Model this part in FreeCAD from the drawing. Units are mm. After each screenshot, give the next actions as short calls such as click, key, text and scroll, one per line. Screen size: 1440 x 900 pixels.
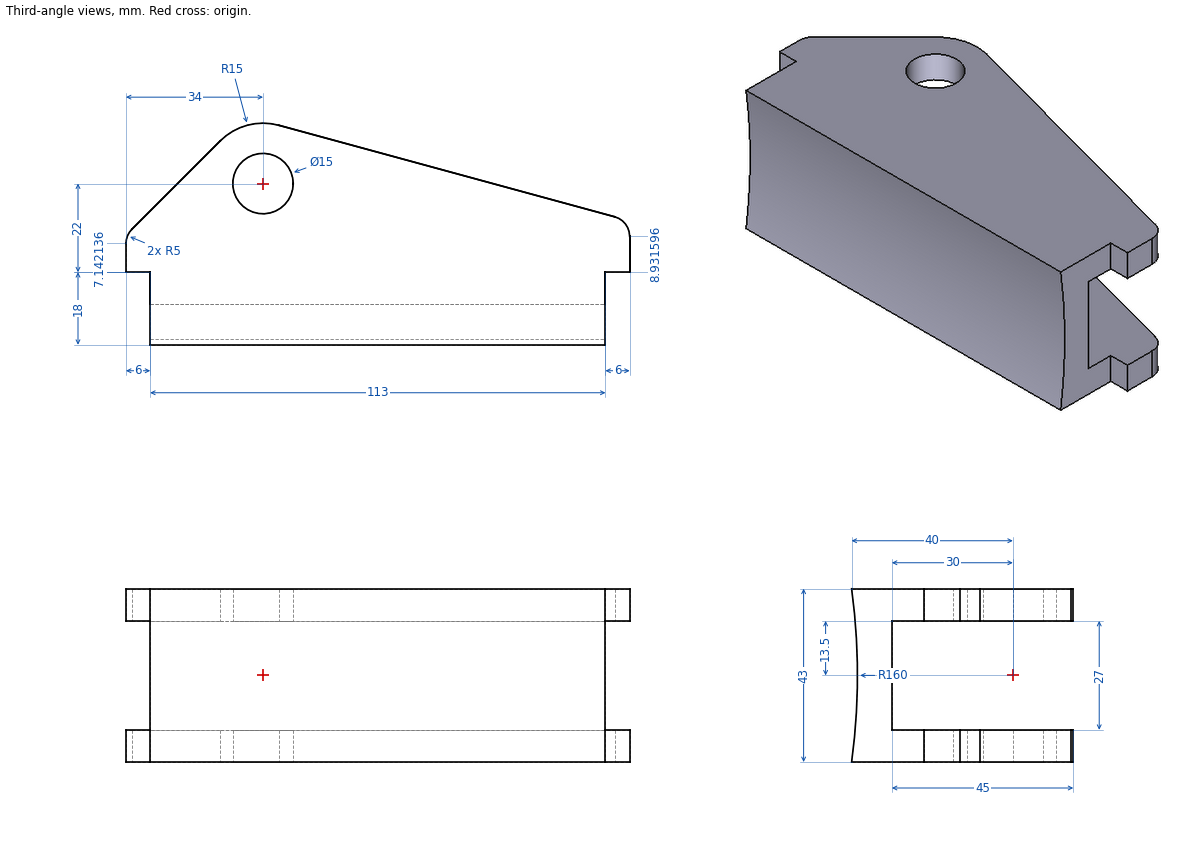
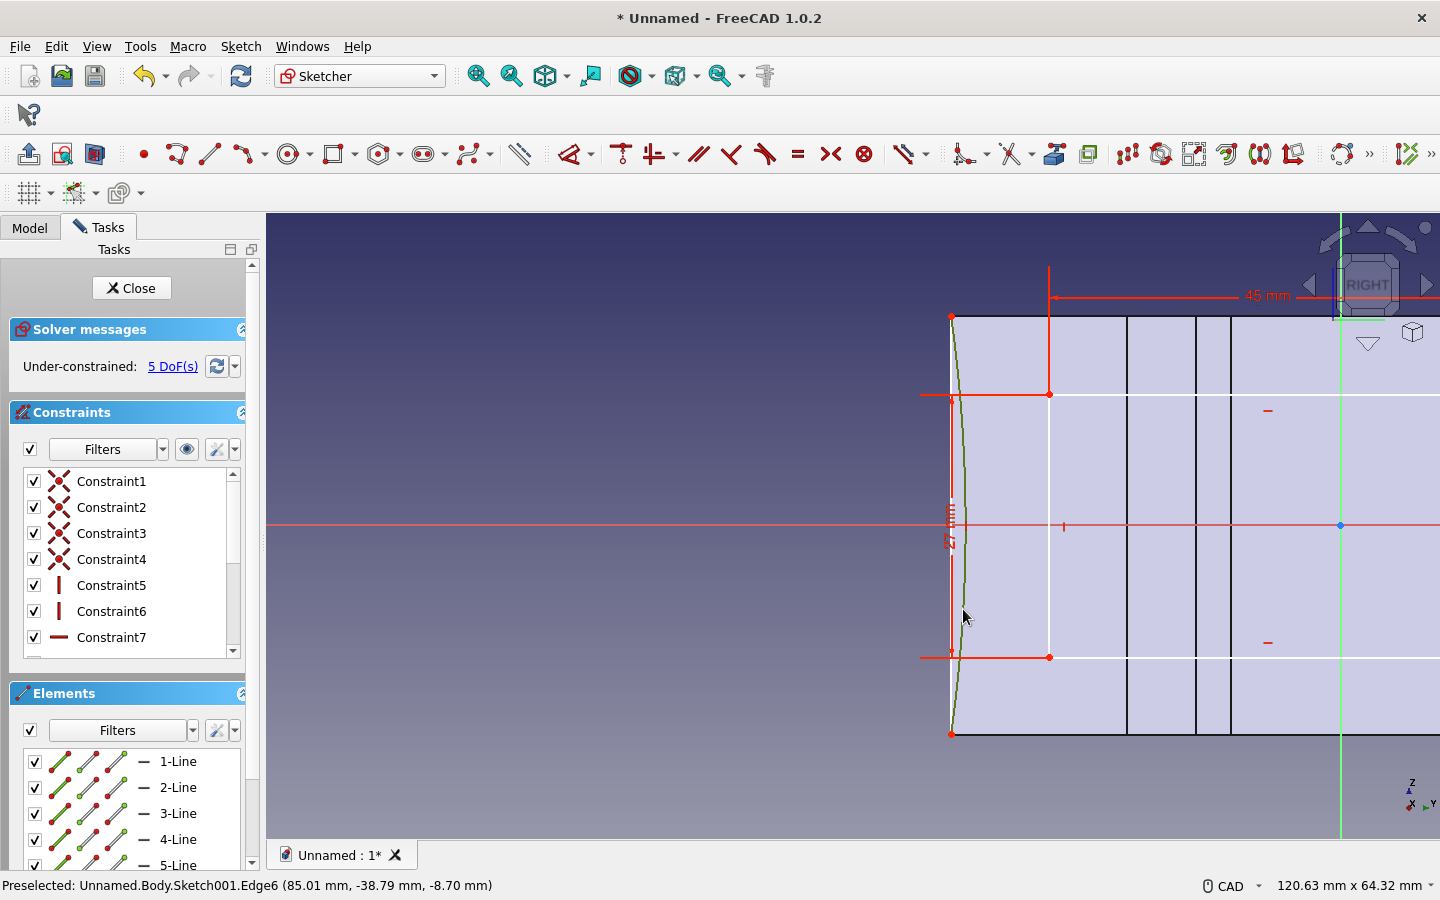
key(k)
key(r)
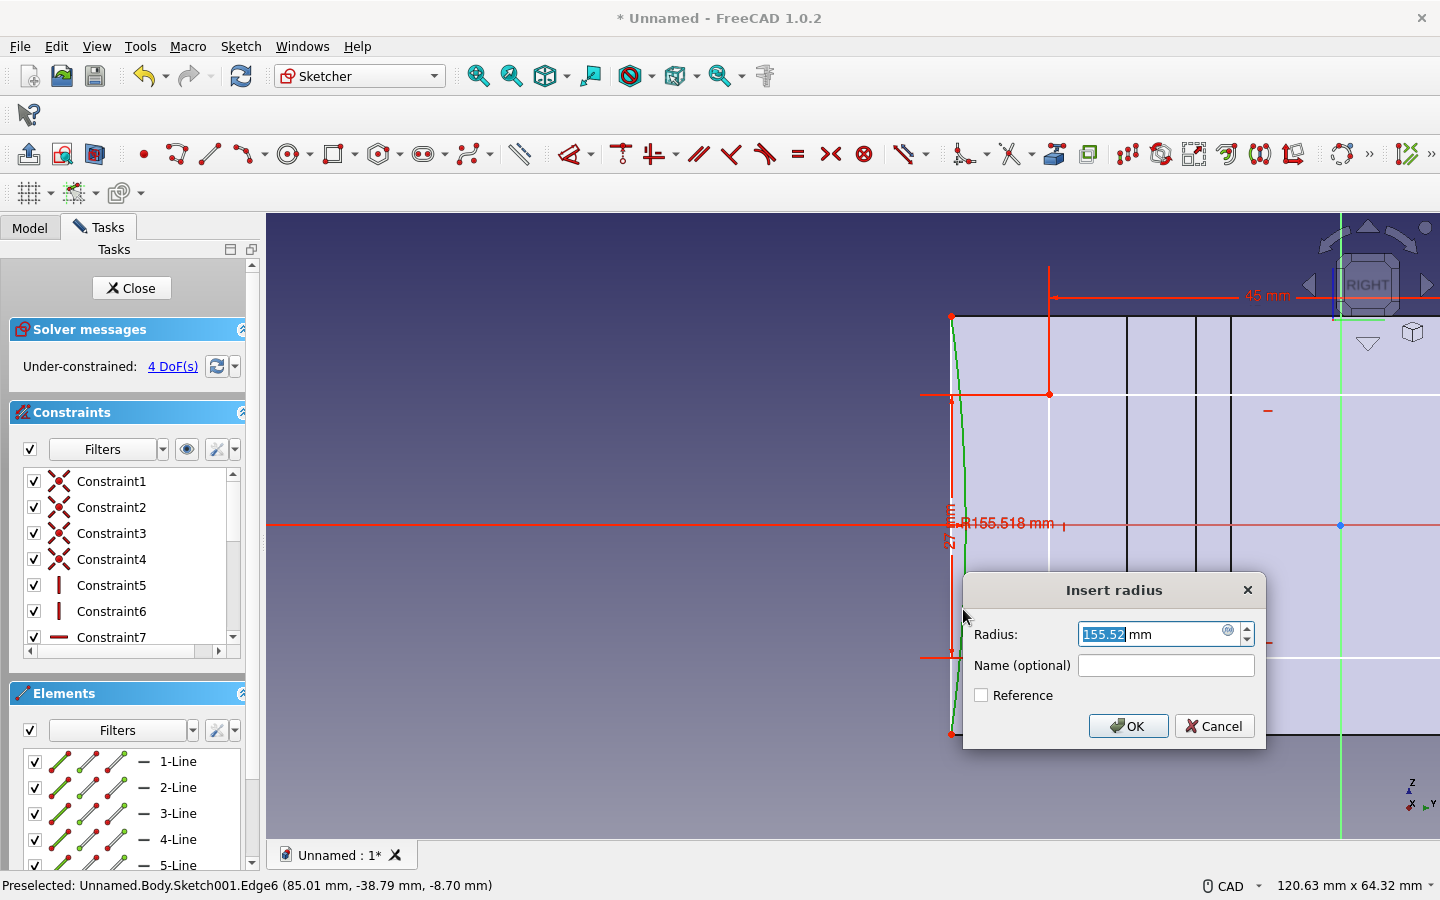
text(160)
key(Return)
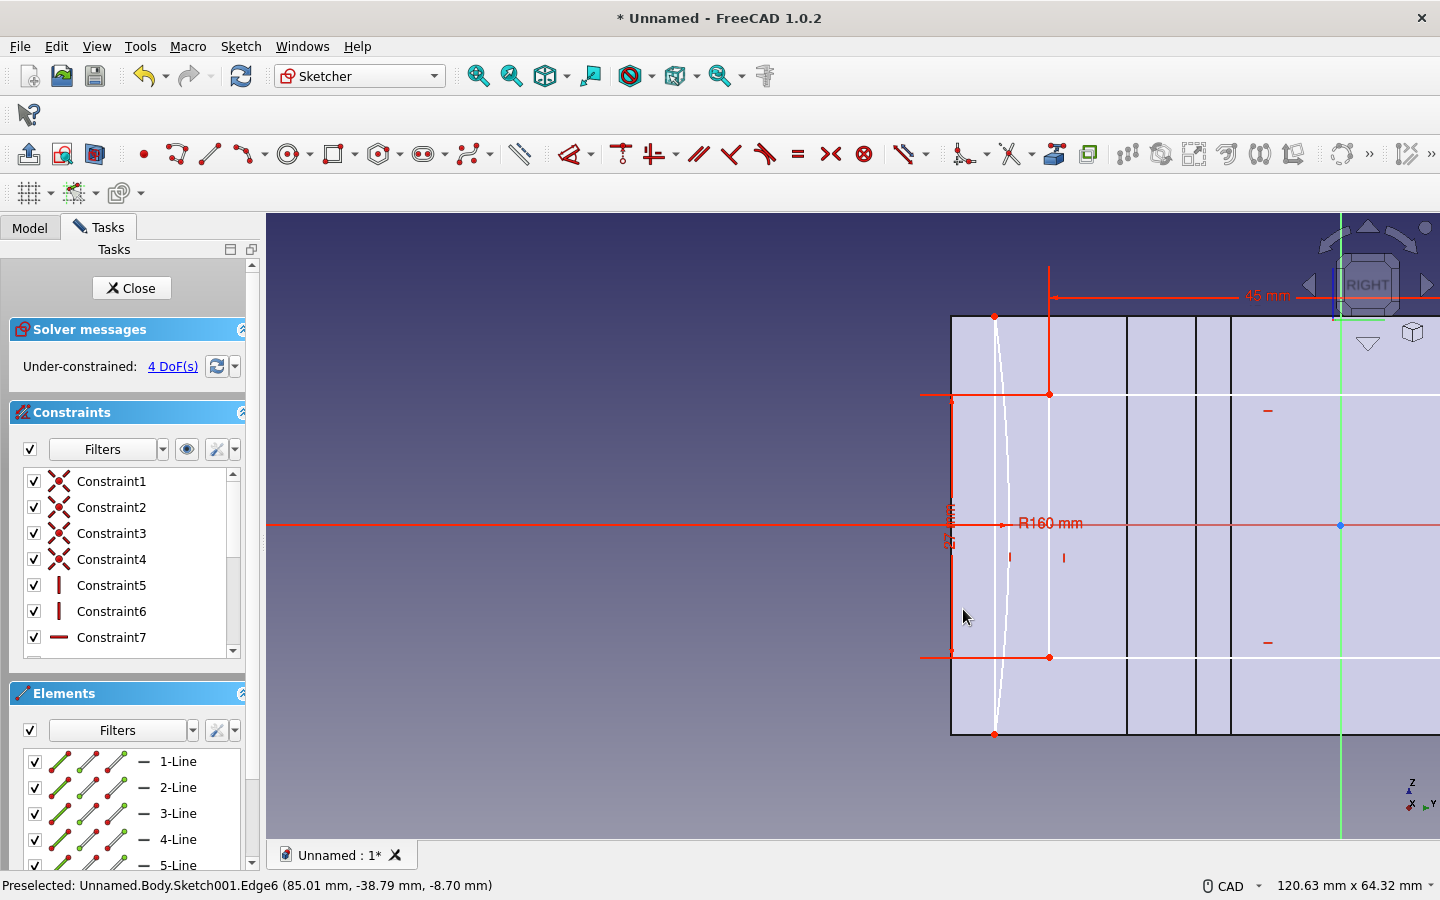
click(995, 442)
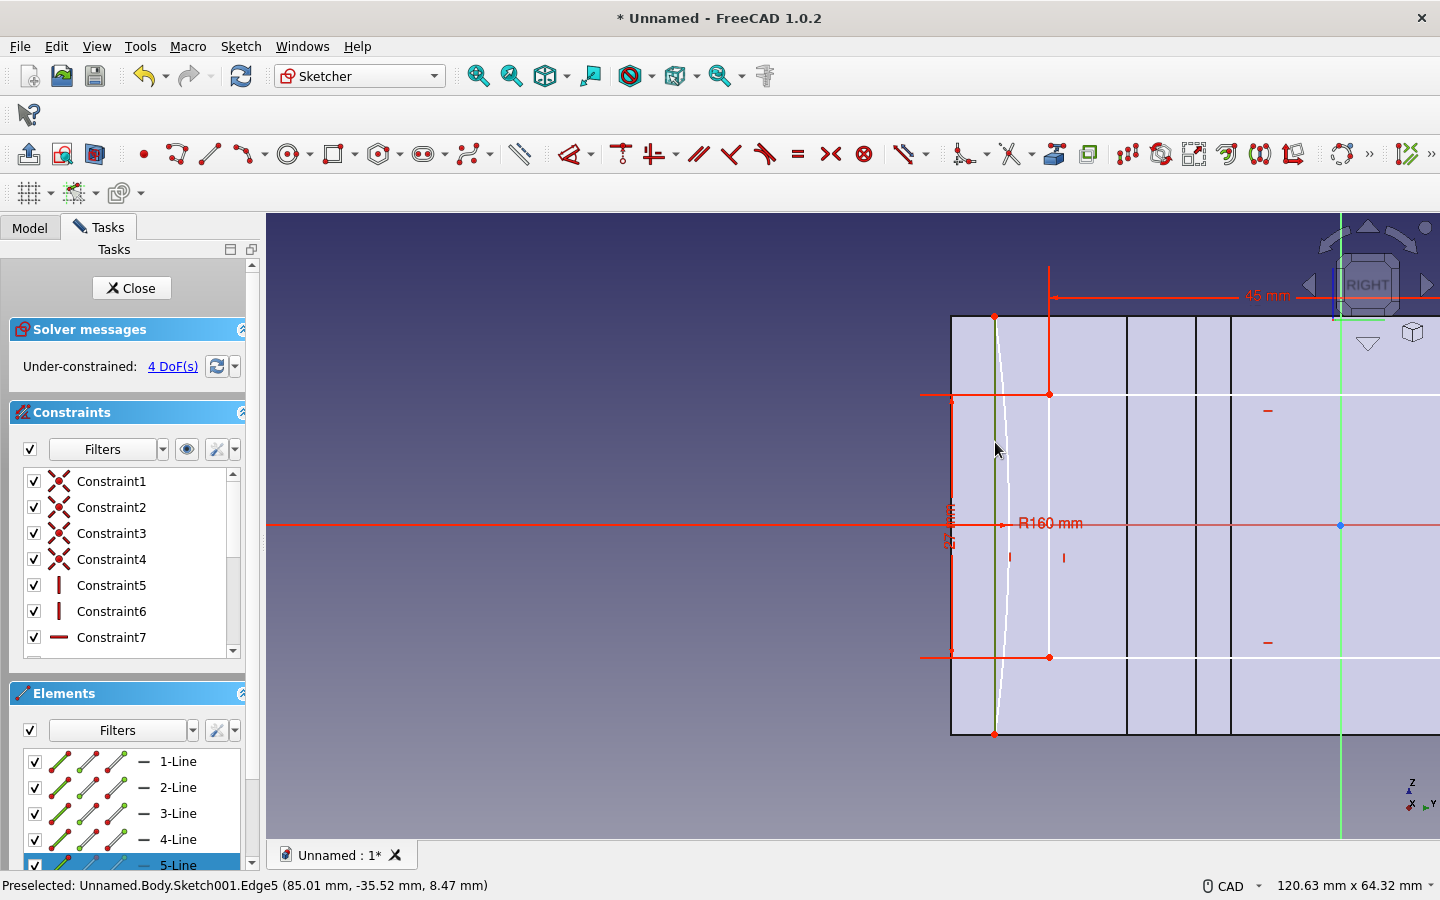
key(i)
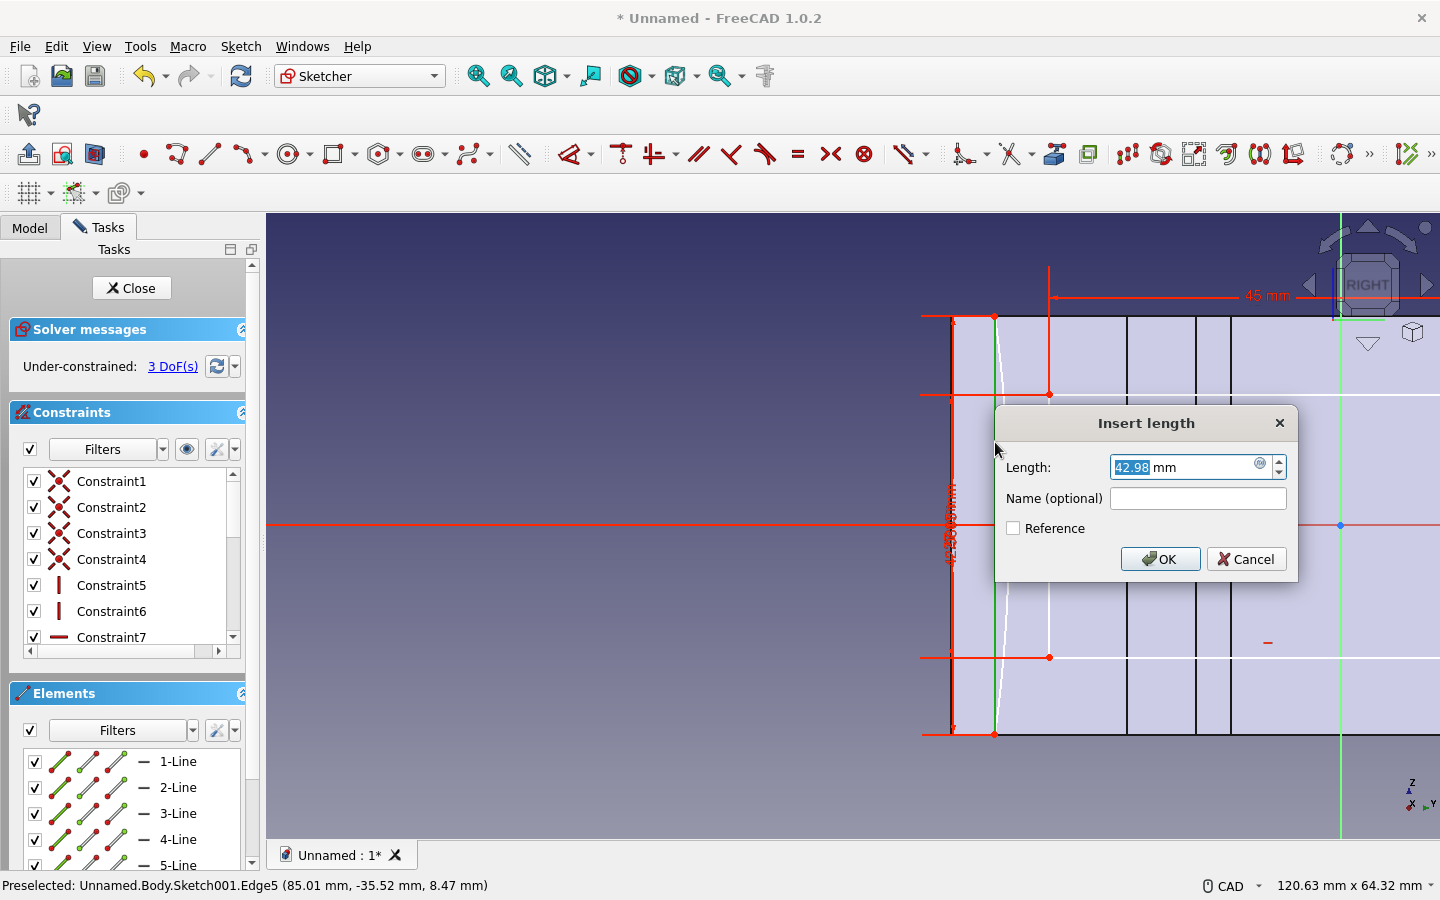
text(43)
key(Return)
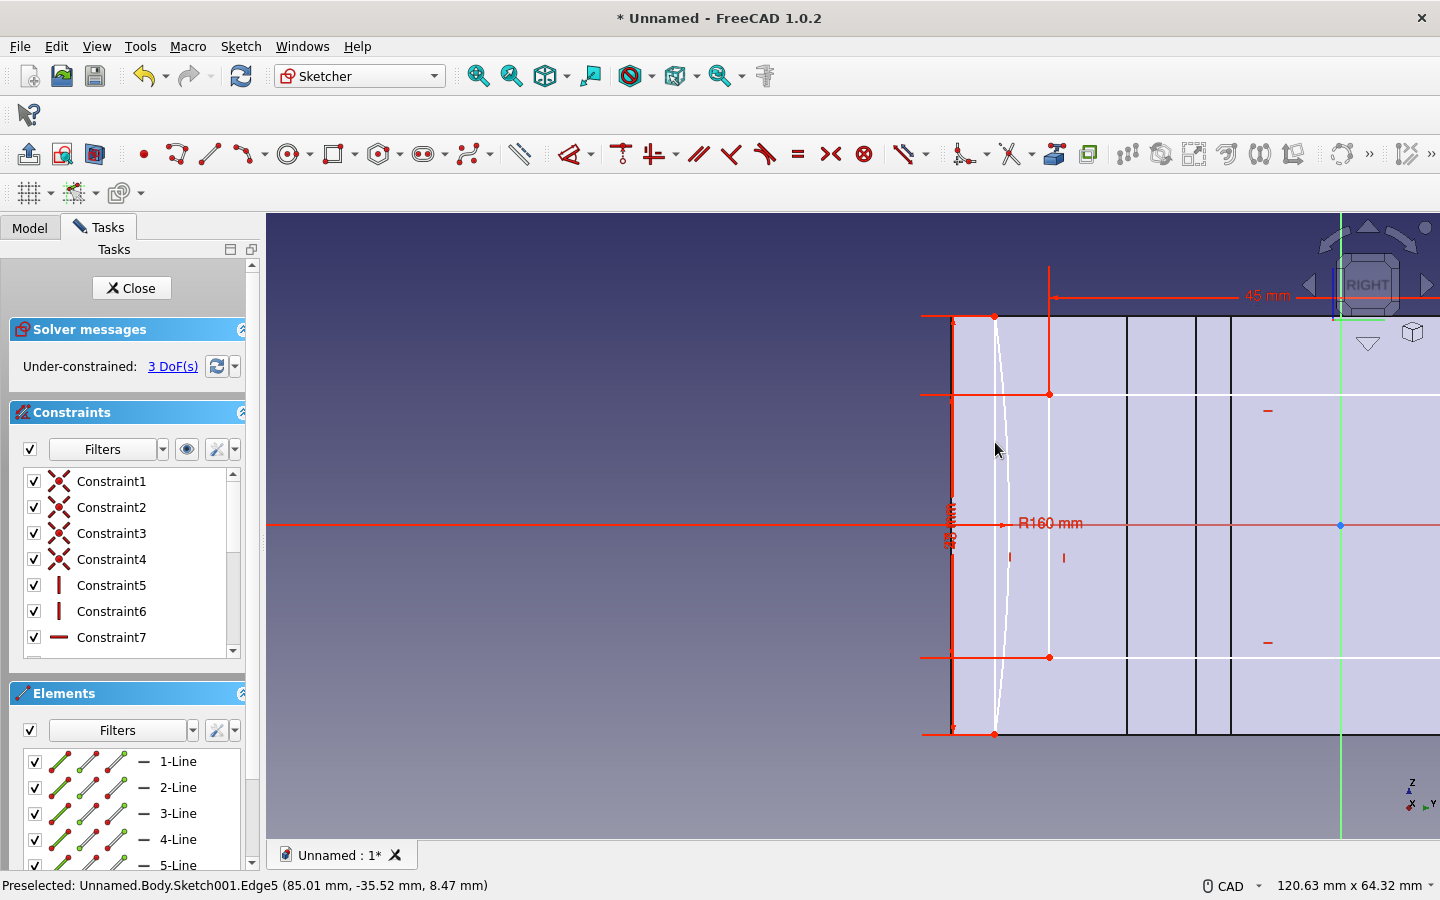
click(1049, 395)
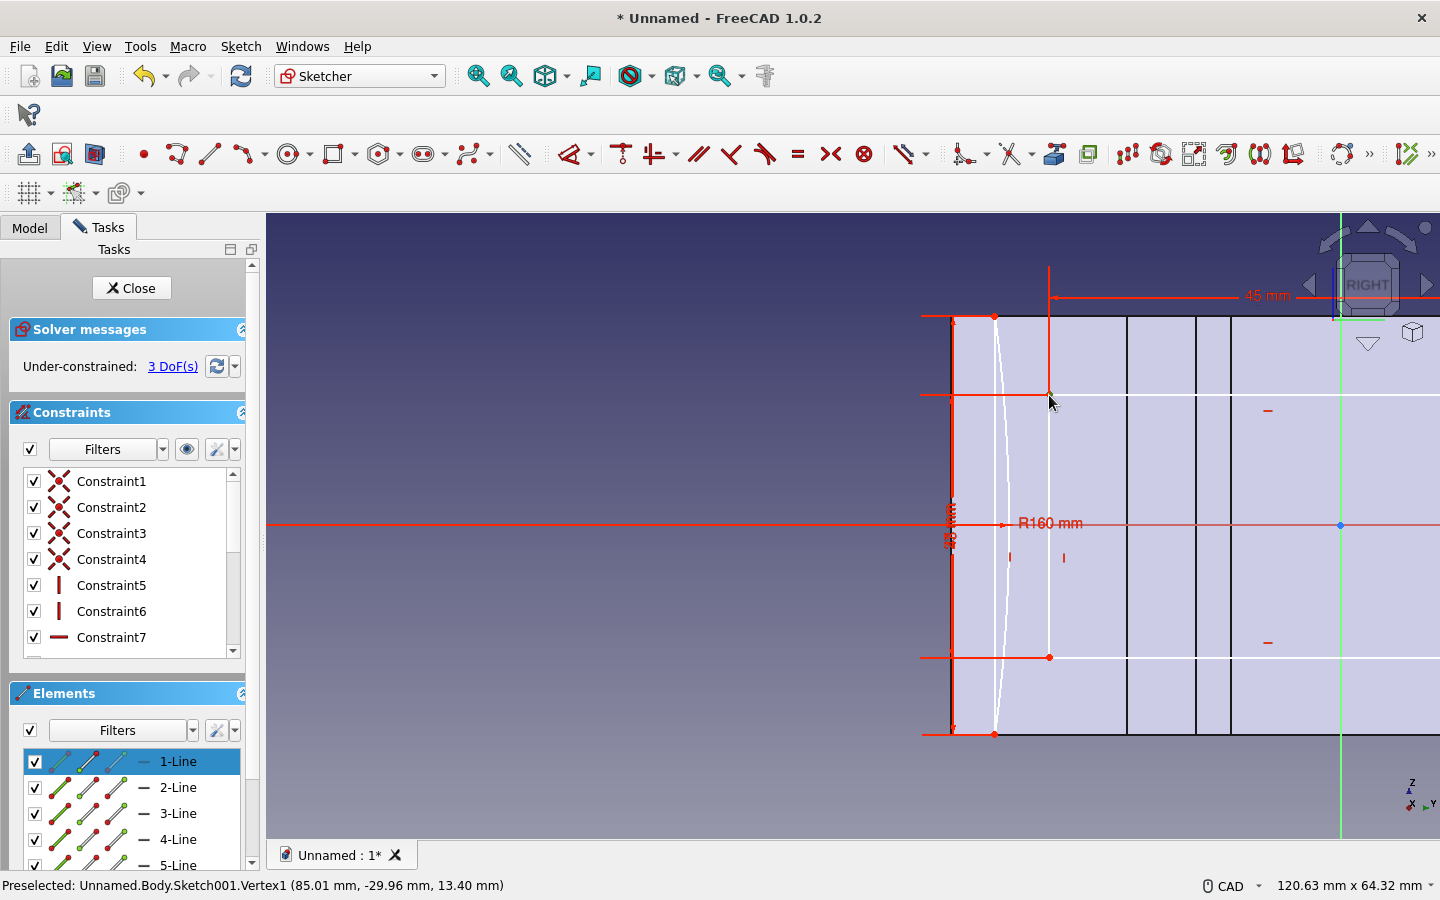
key(l)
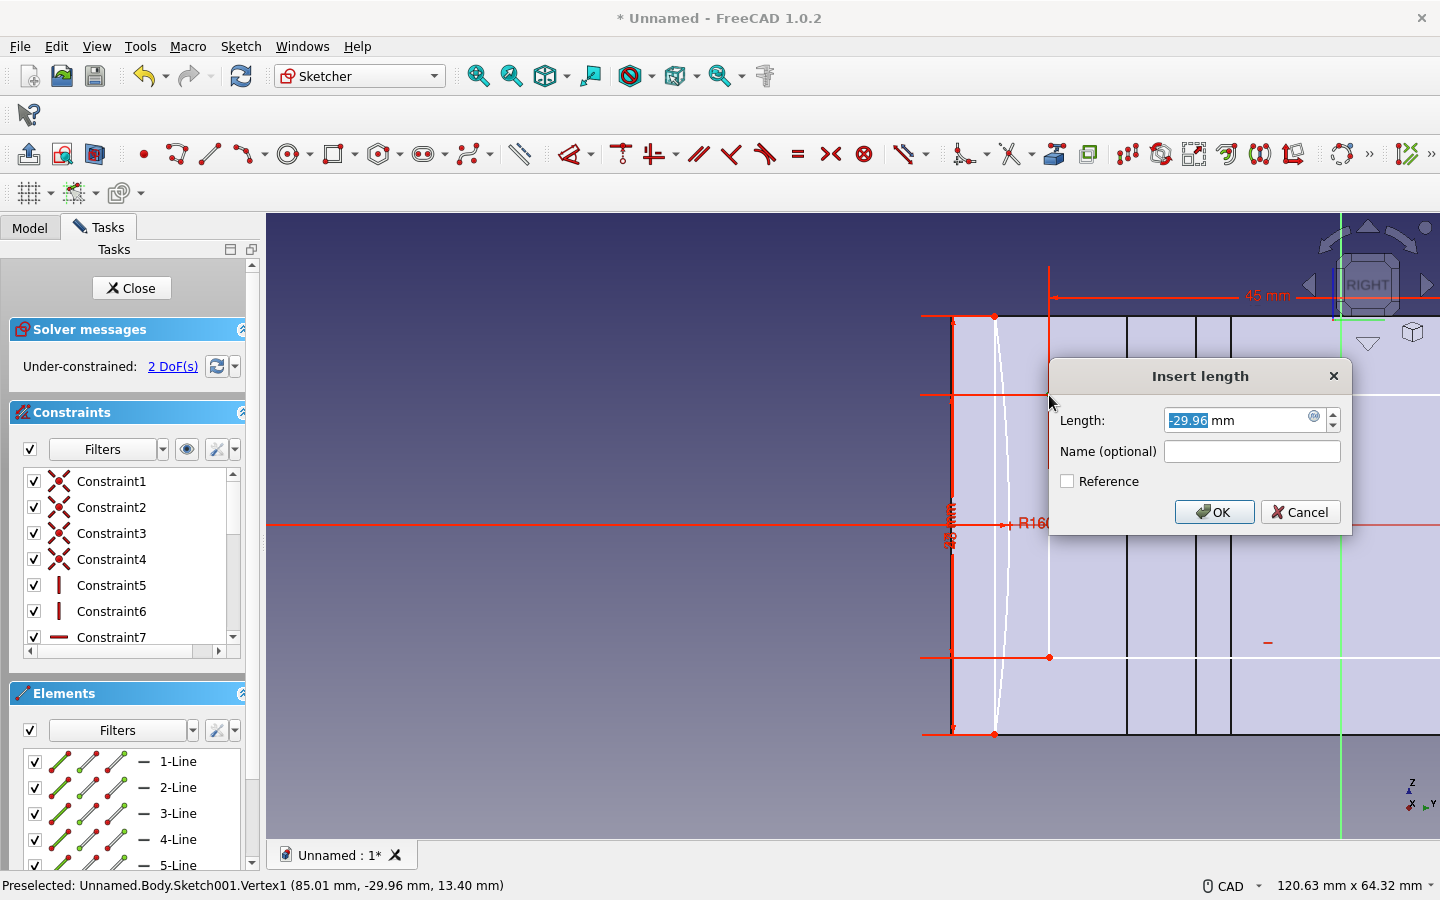
text(-30)
key(Return)